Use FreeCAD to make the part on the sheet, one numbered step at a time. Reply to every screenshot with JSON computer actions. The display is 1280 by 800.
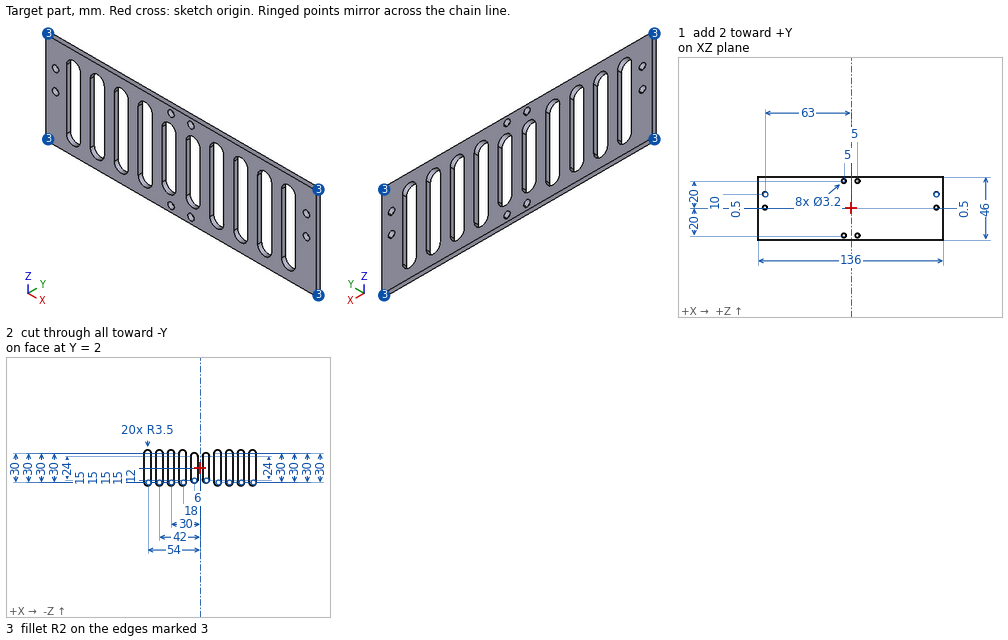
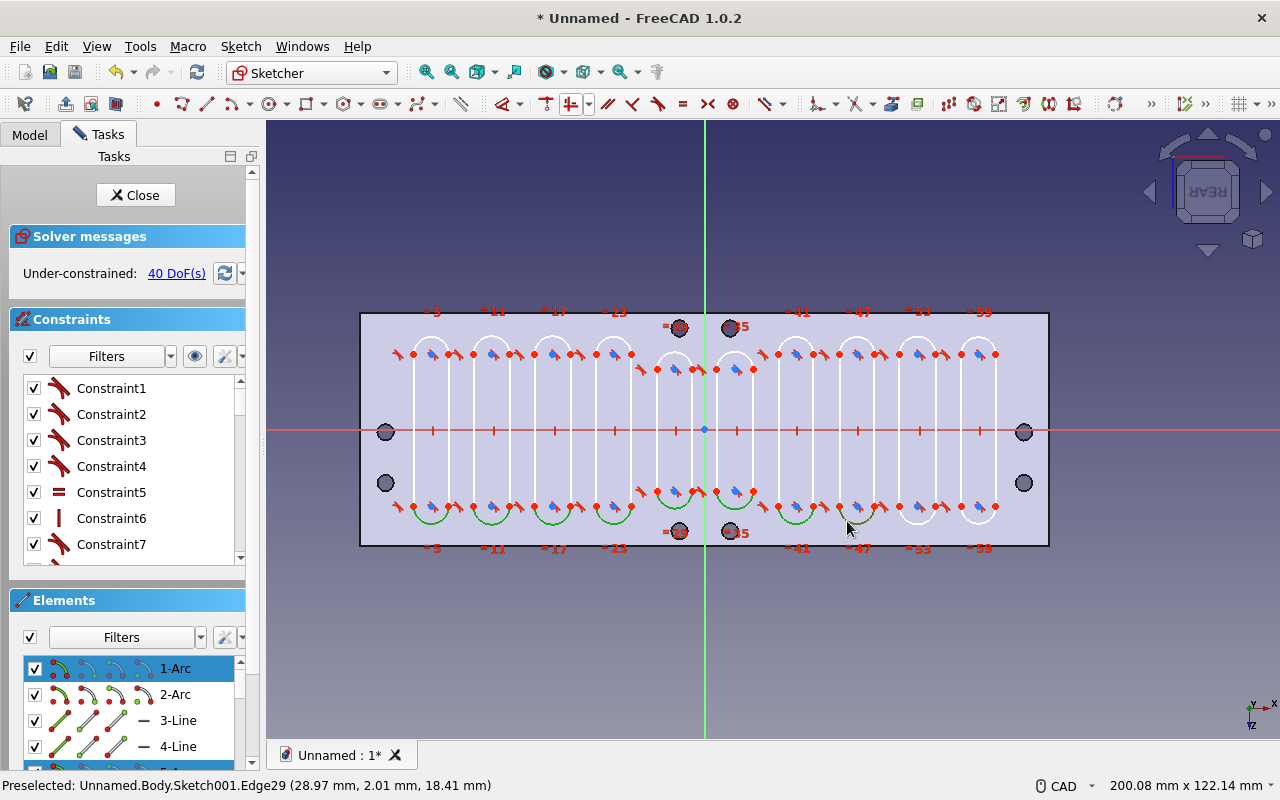
{"action": "left_click", "coordinate": [907, 521]}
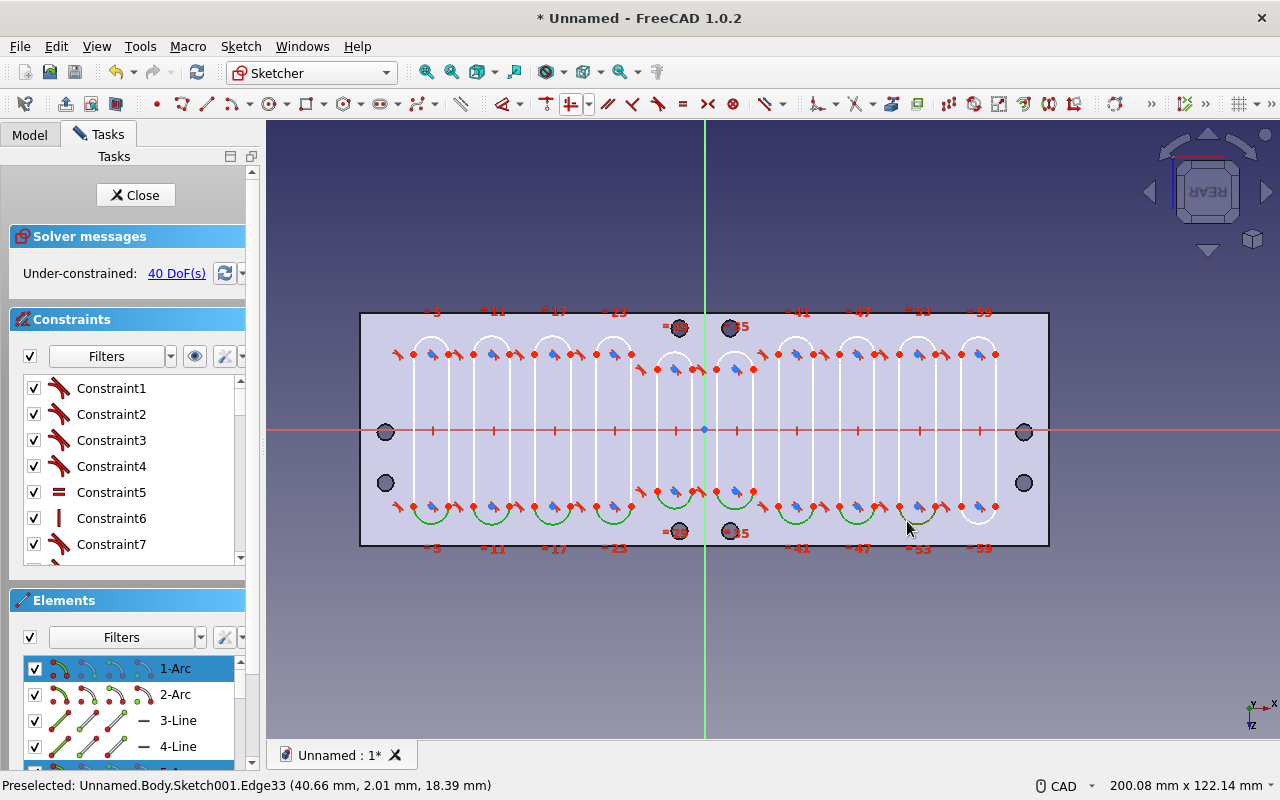
{"action": "left_click", "coordinate": [968, 520]}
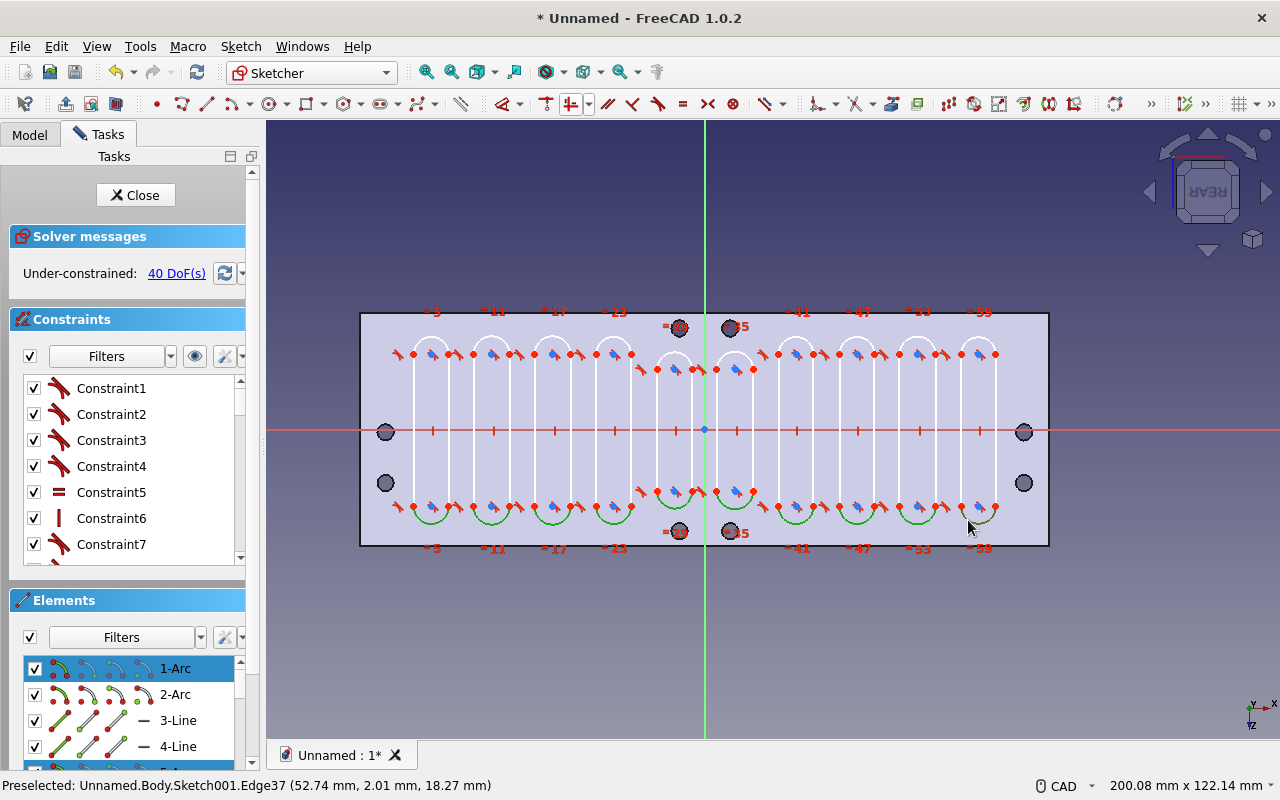
{"action": "left_click", "coordinate": [683, 104]}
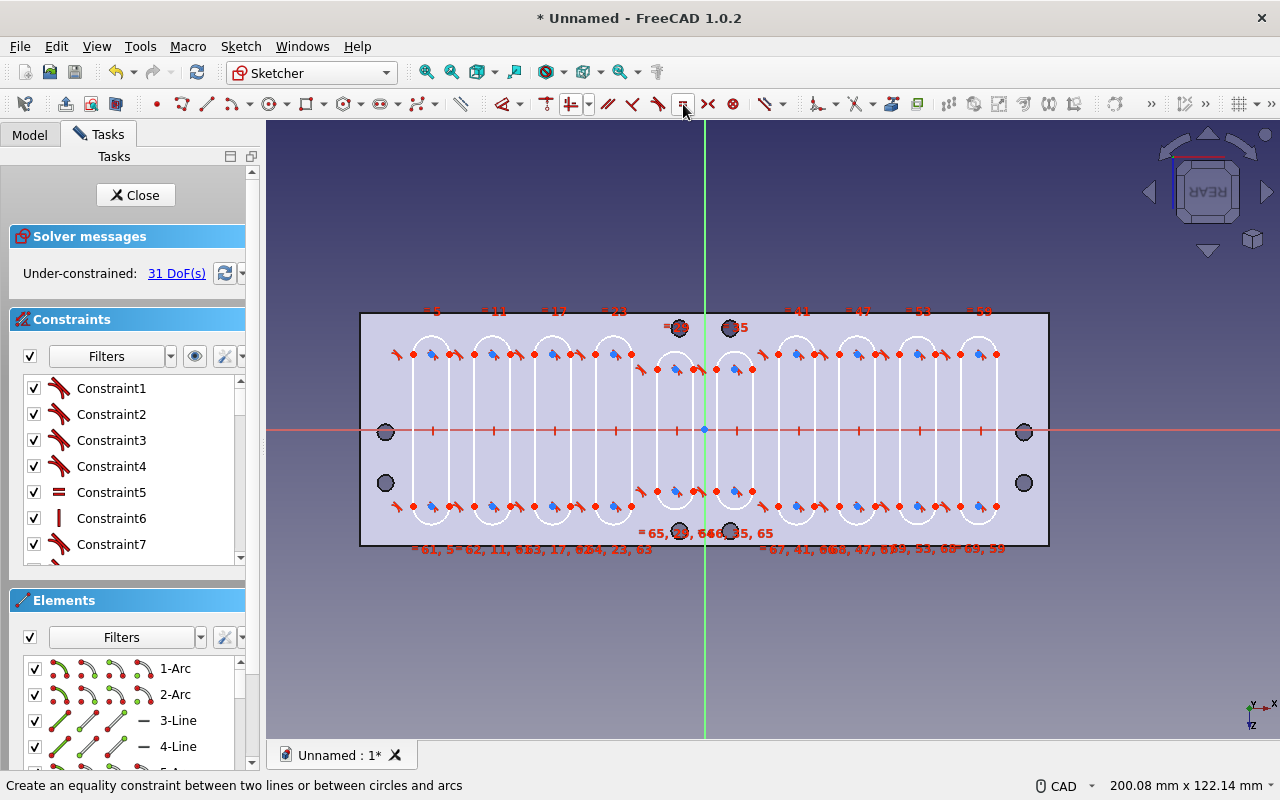
{"action": "left_click", "coordinate": [675, 491]}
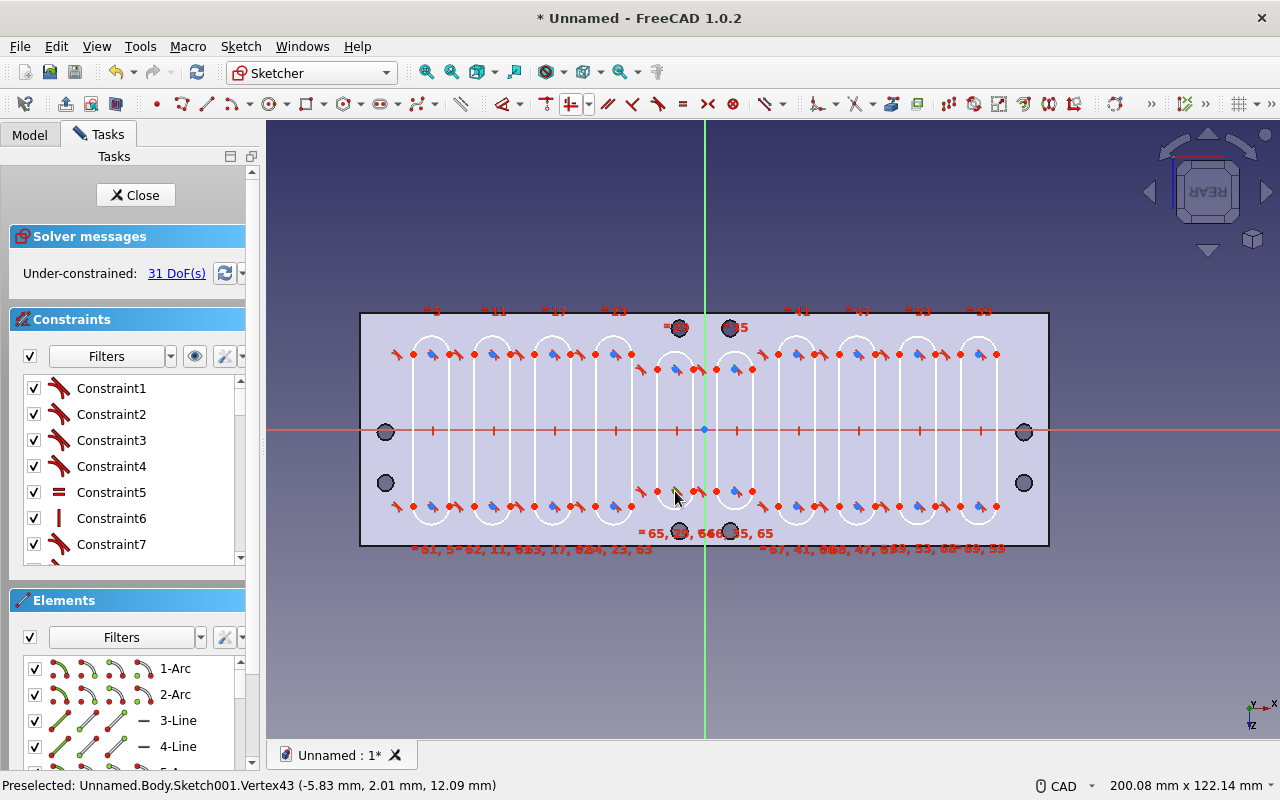
{"action": "left_click", "coordinate": [735, 491]}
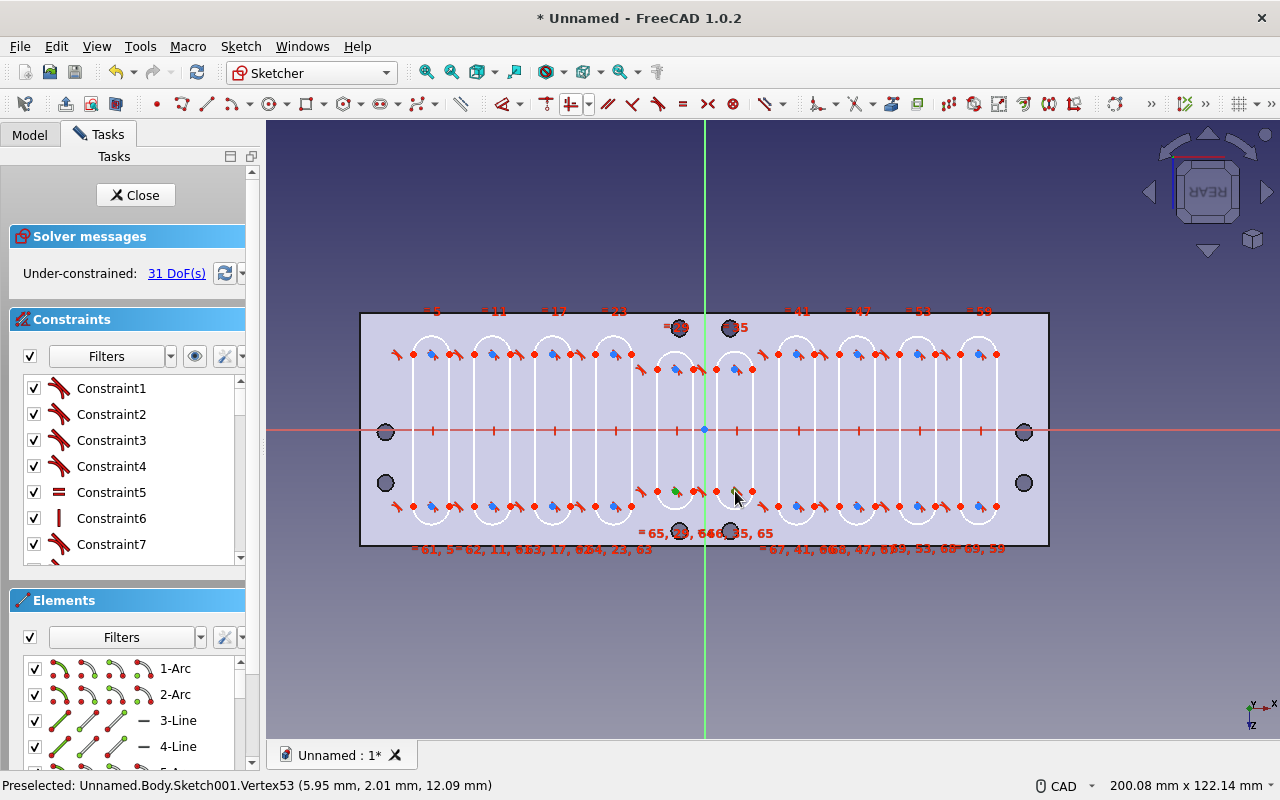
{"action": "left_click", "coordinate": [705, 671]}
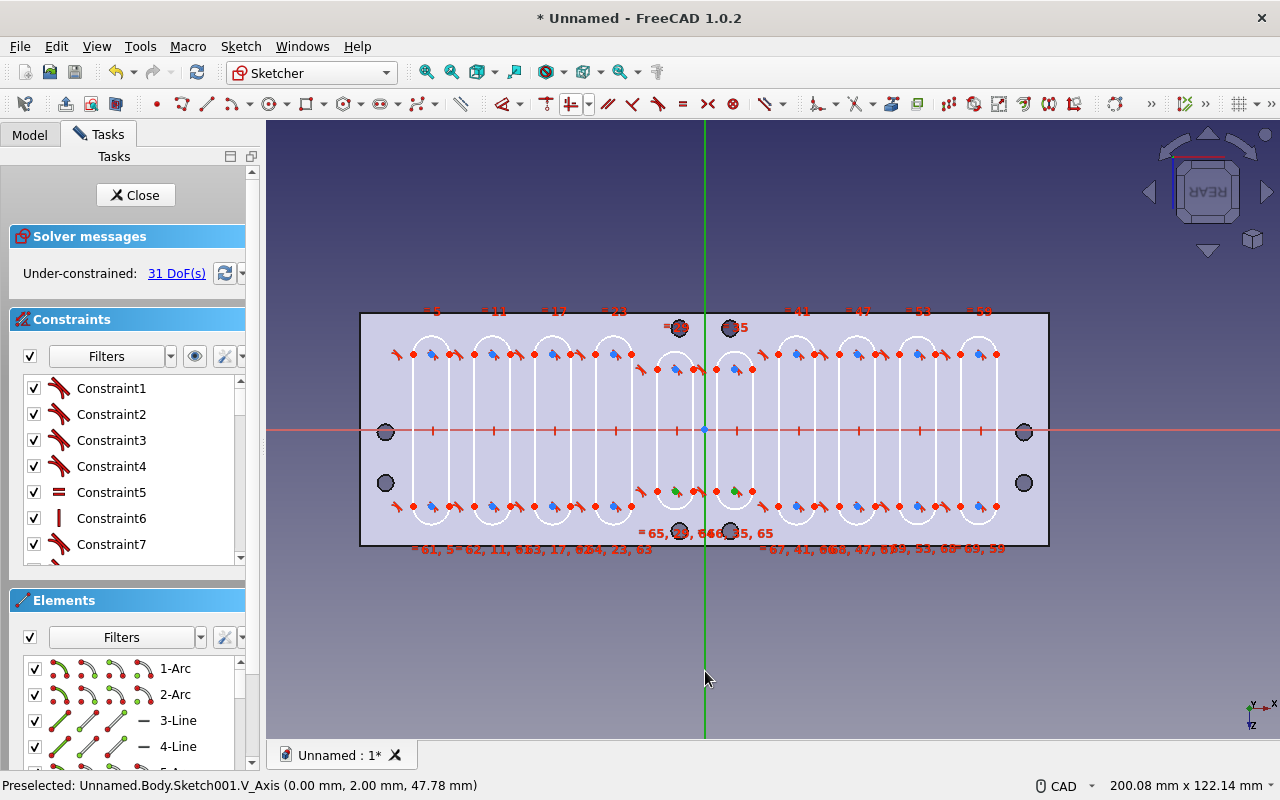
{"action": "left_click", "coordinate": [708, 104]}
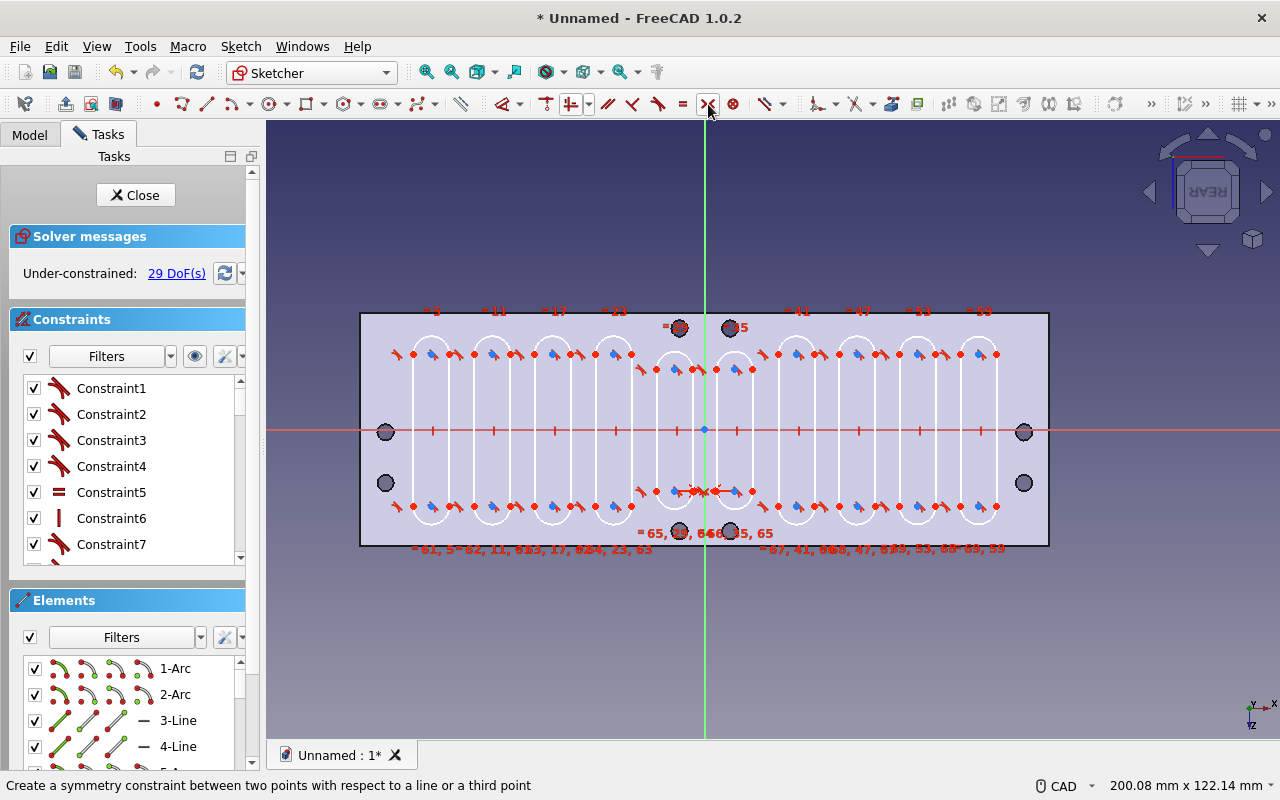
{"action": "left_click", "coordinate": [614, 507]}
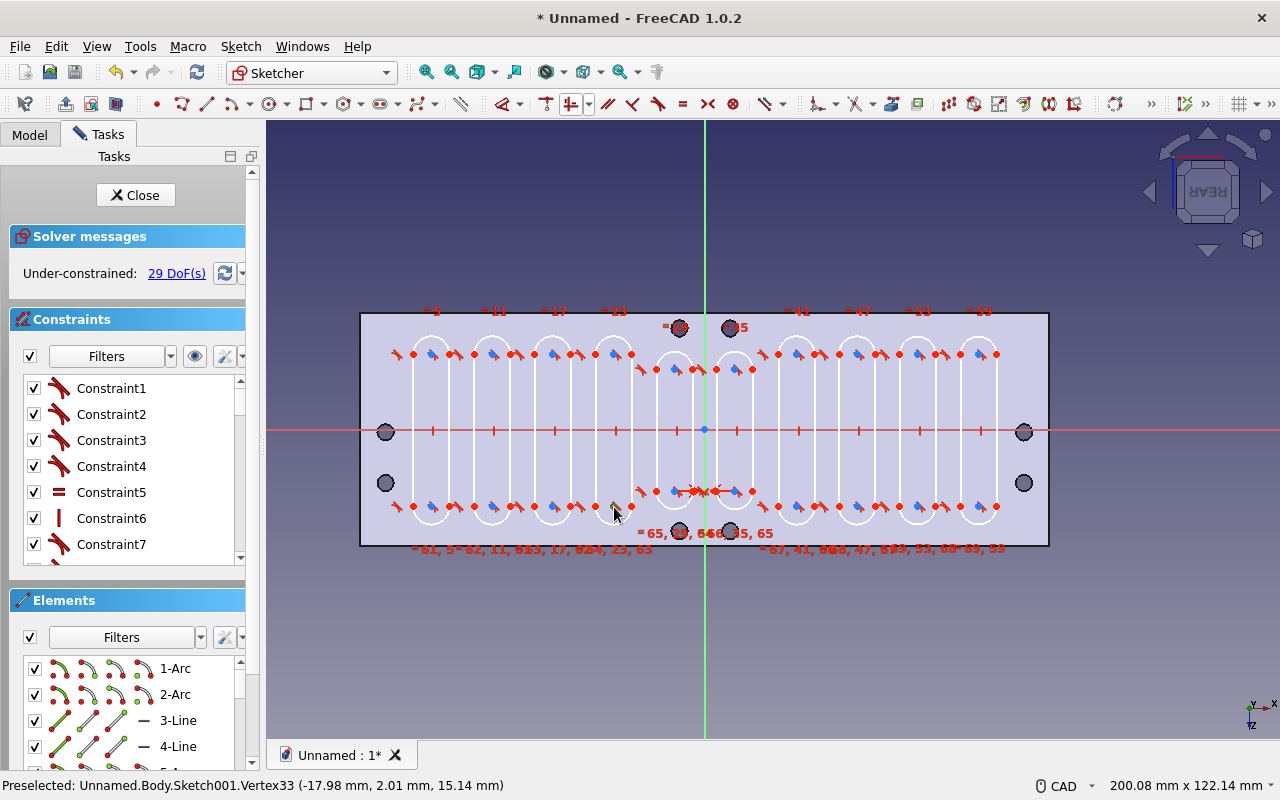
{"action": "left_click", "coordinate": [797, 507]}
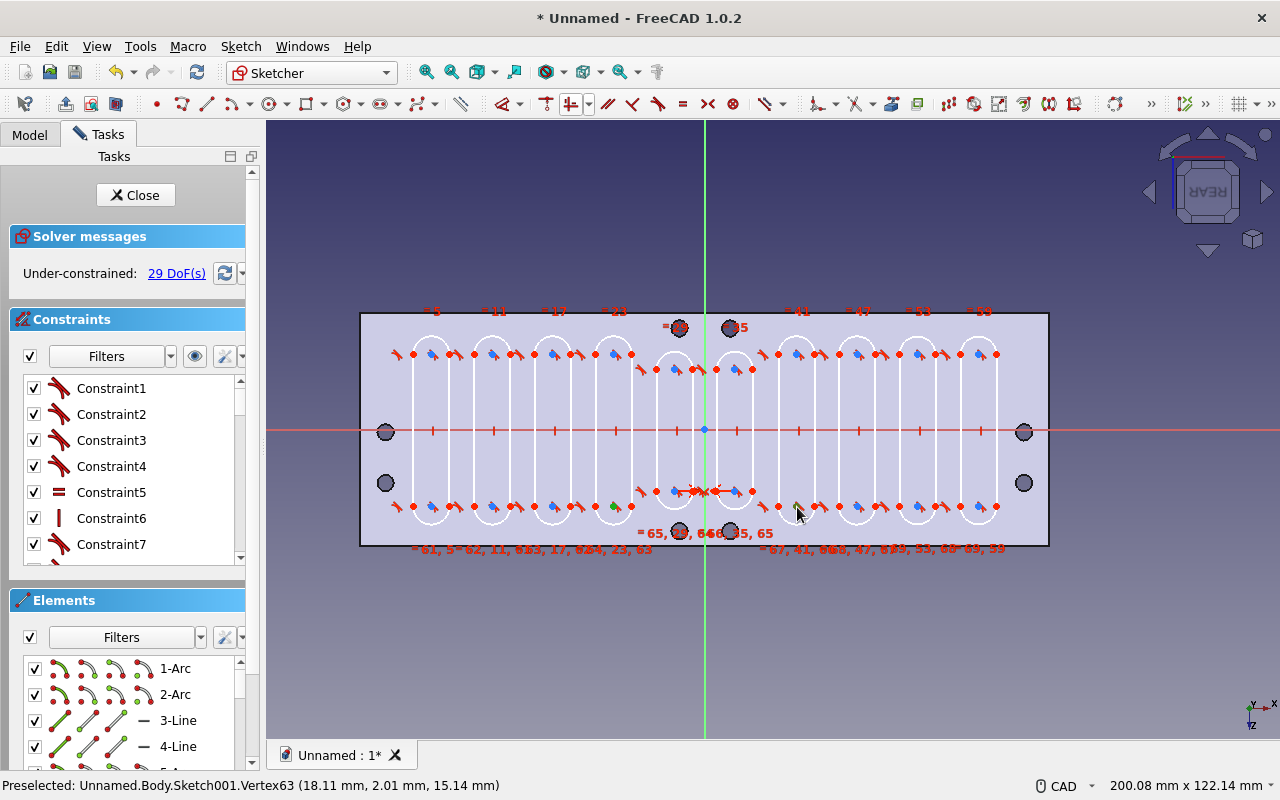
{"action": "left_click", "coordinate": [705, 671]}